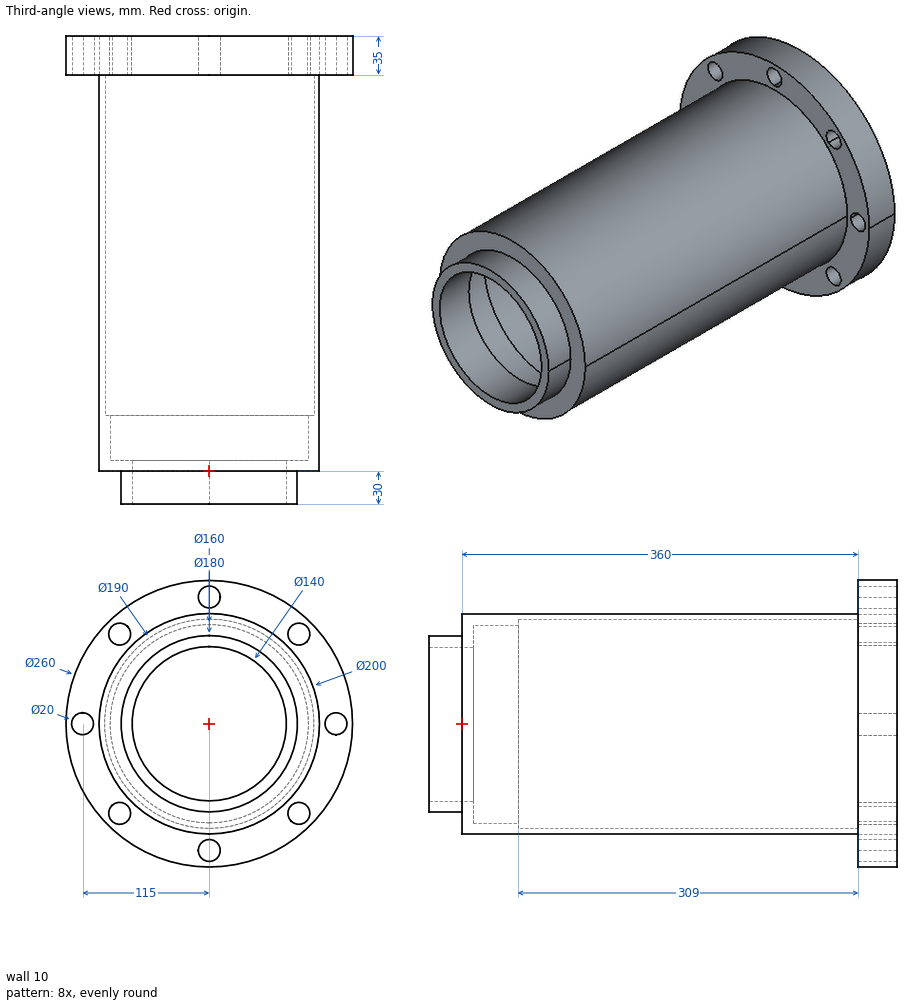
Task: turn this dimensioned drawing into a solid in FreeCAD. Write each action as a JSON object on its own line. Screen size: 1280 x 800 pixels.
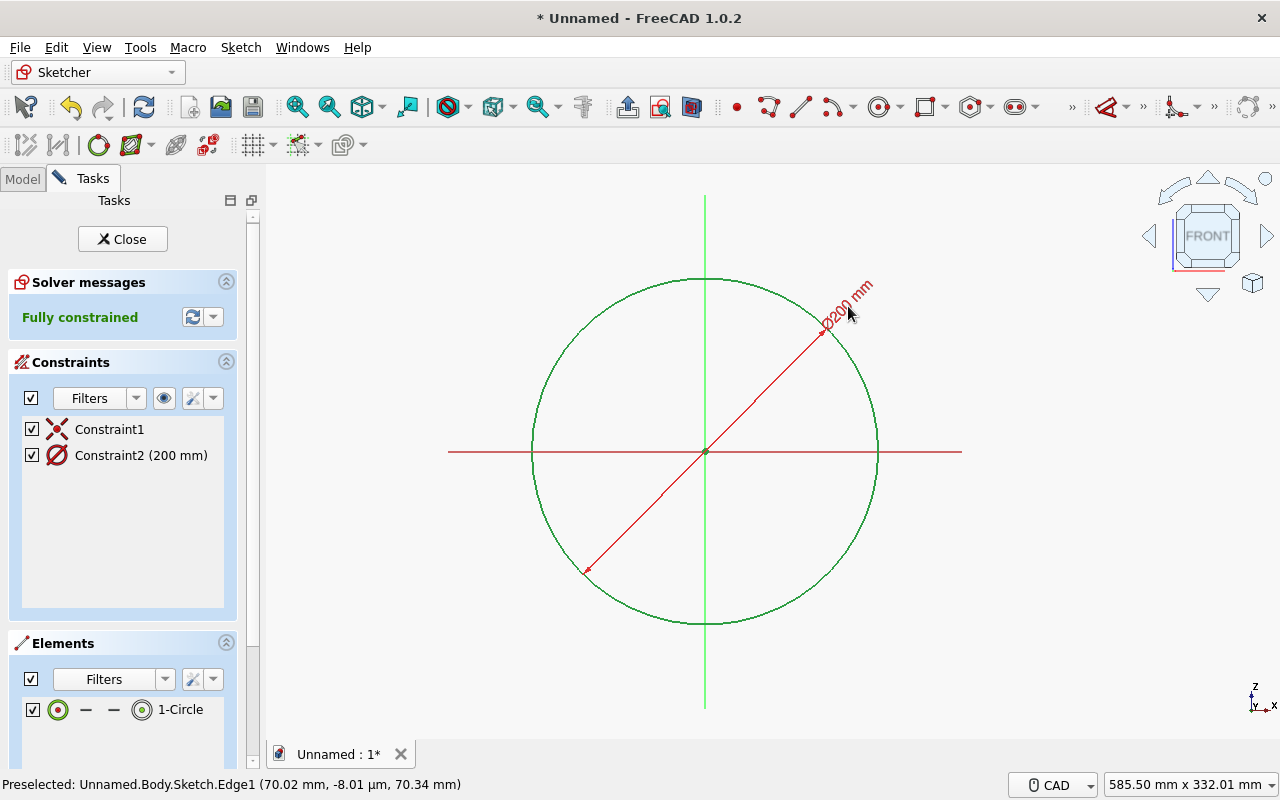
{"action": "left_click", "coordinate": [123, 239]}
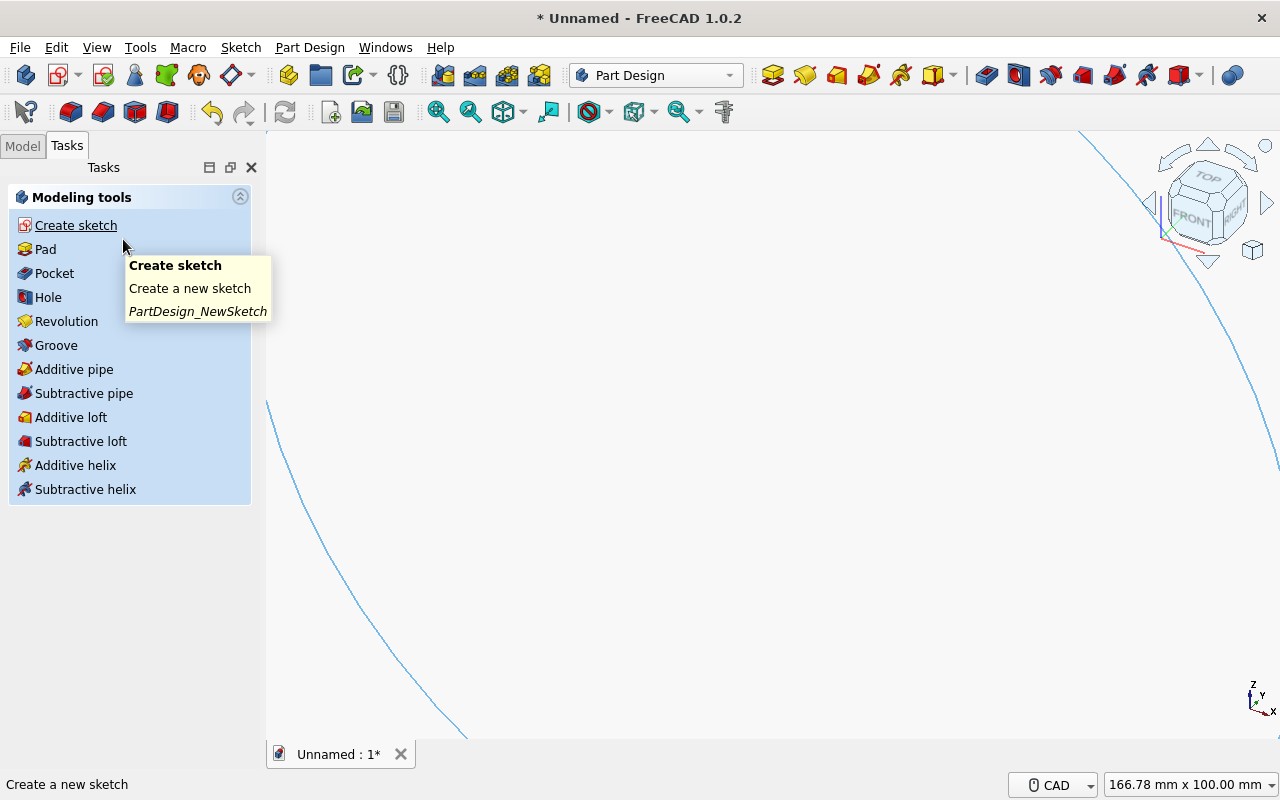
{"action": "left_click", "coordinate": [774, 76]}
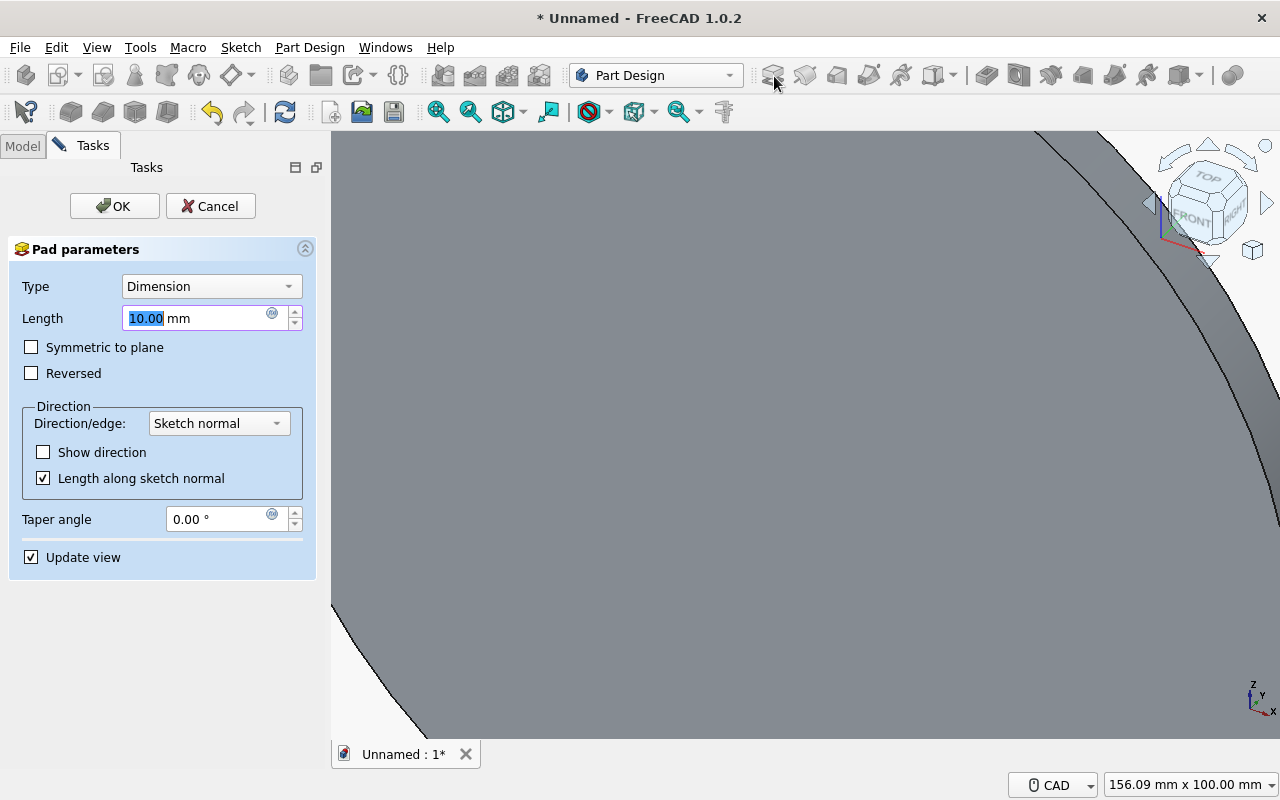
{"action": "type", "text": "360"}
{"action": "key", "text": "Tab"}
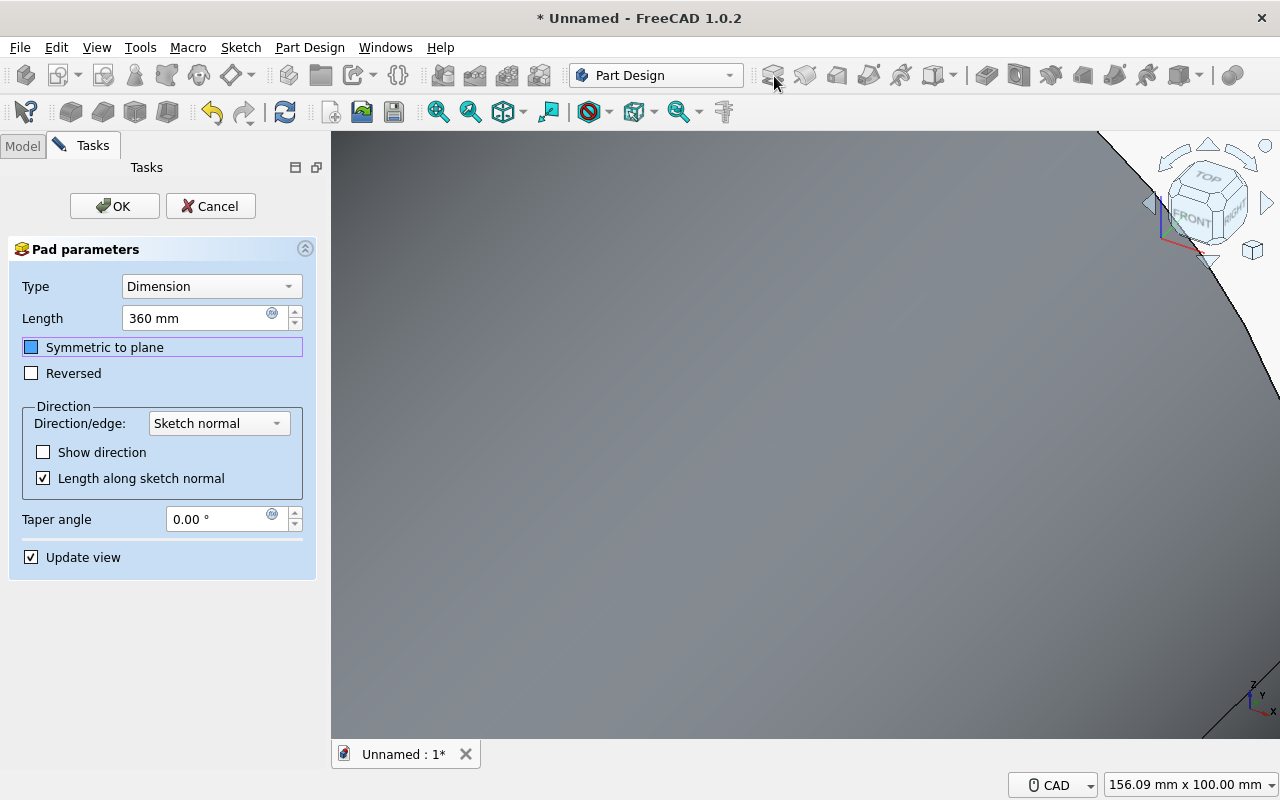
{"action": "left_click", "coordinate": [30, 373]}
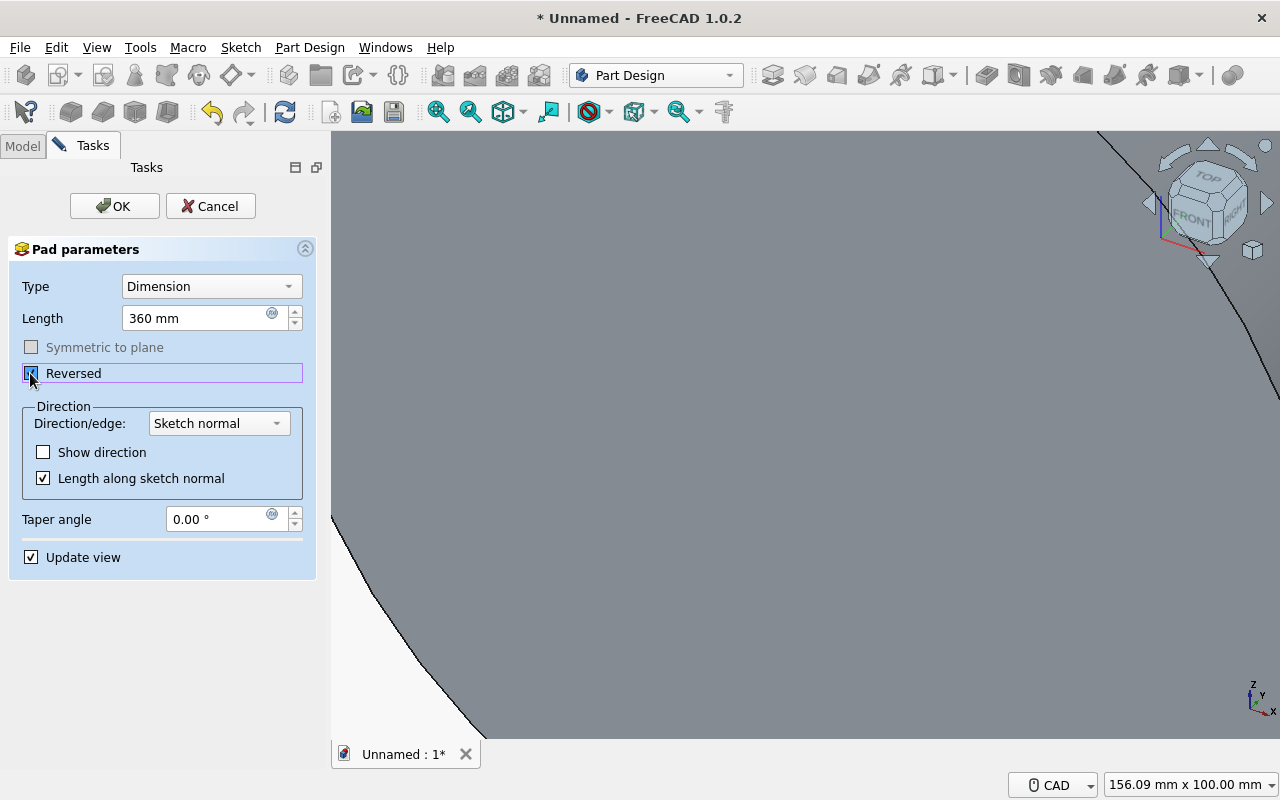
{"action": "left_click", "coordinate": [115, 206]}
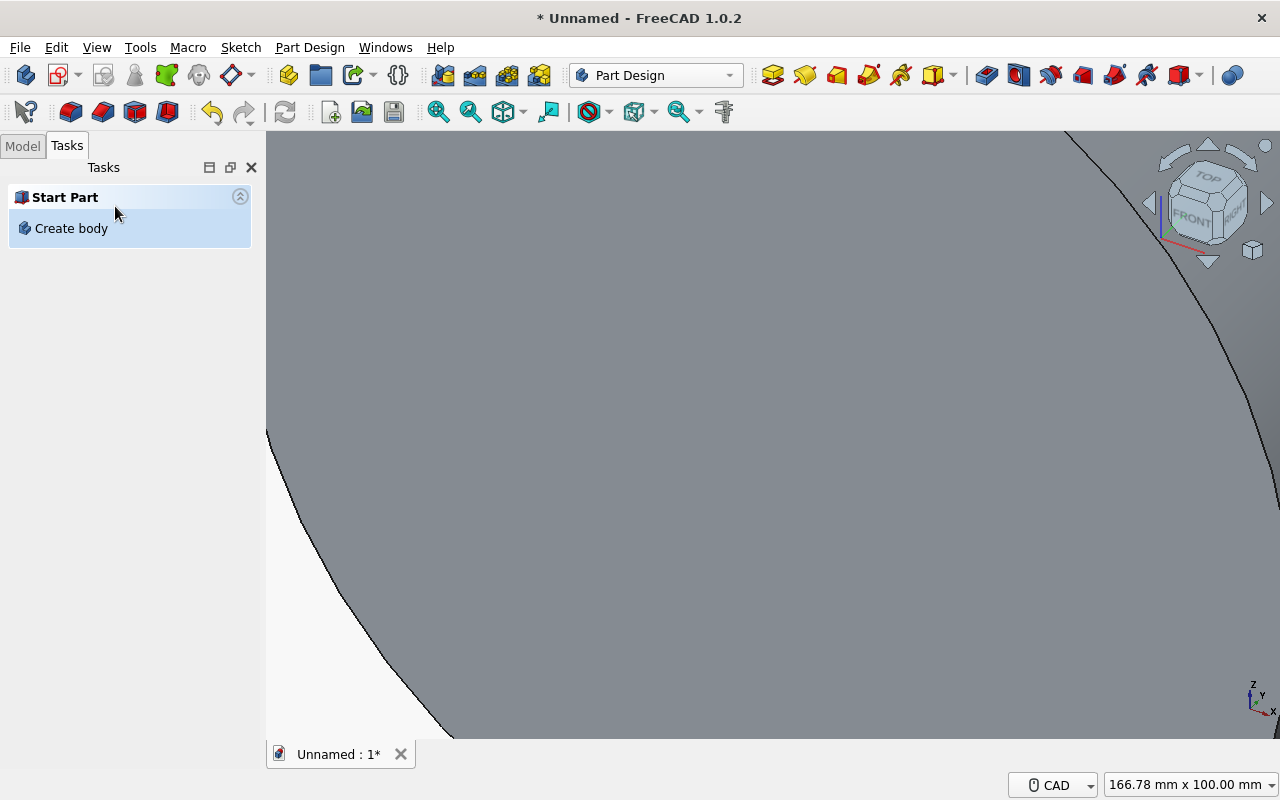
{"action": "left_click", "coordinate": [440, 112]}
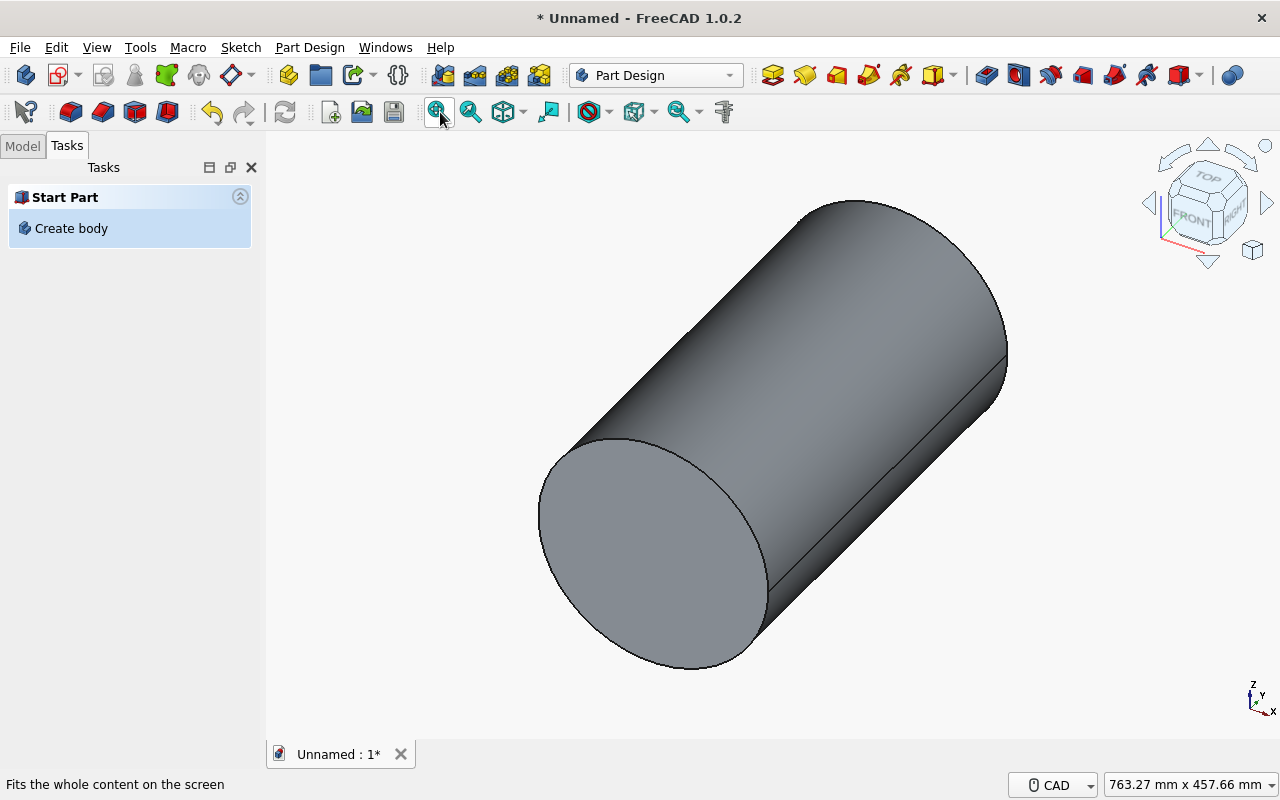
{"action": "key", "text": "0"}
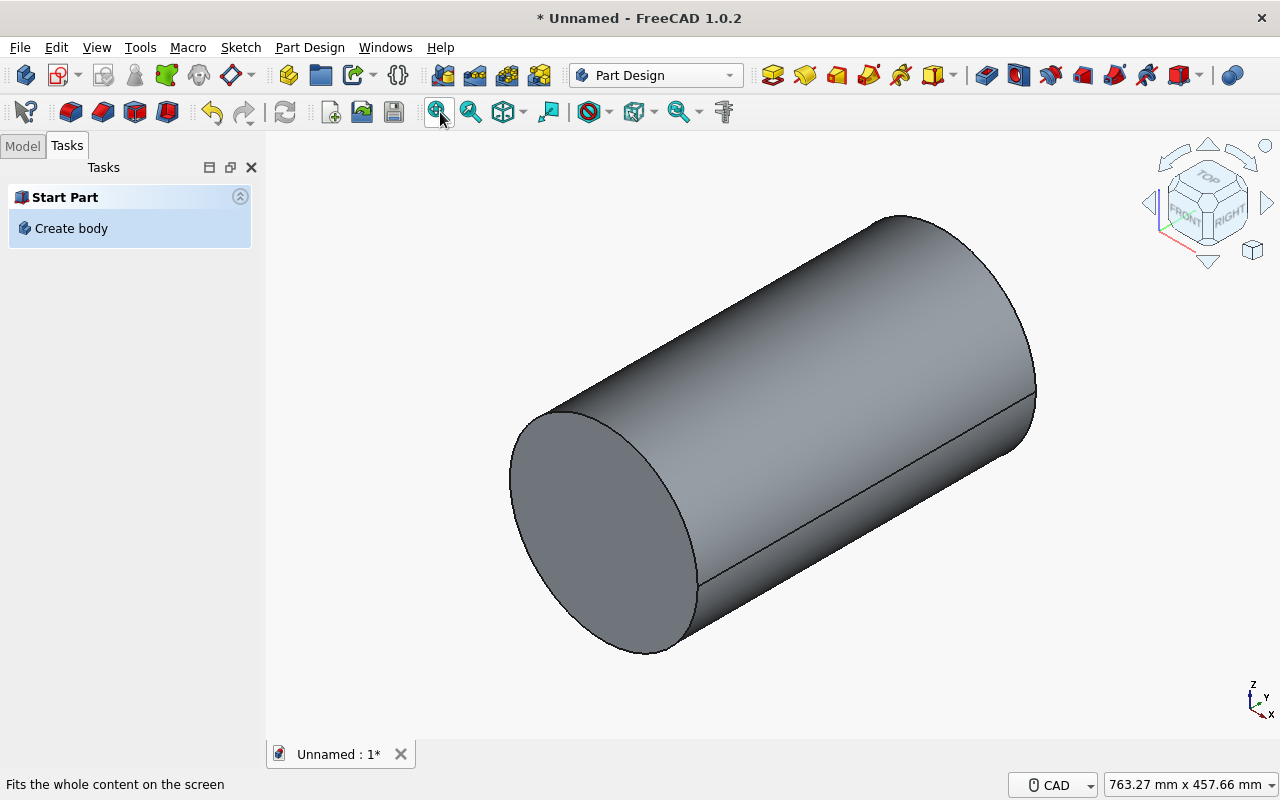
{"action": "key", "text": "2"}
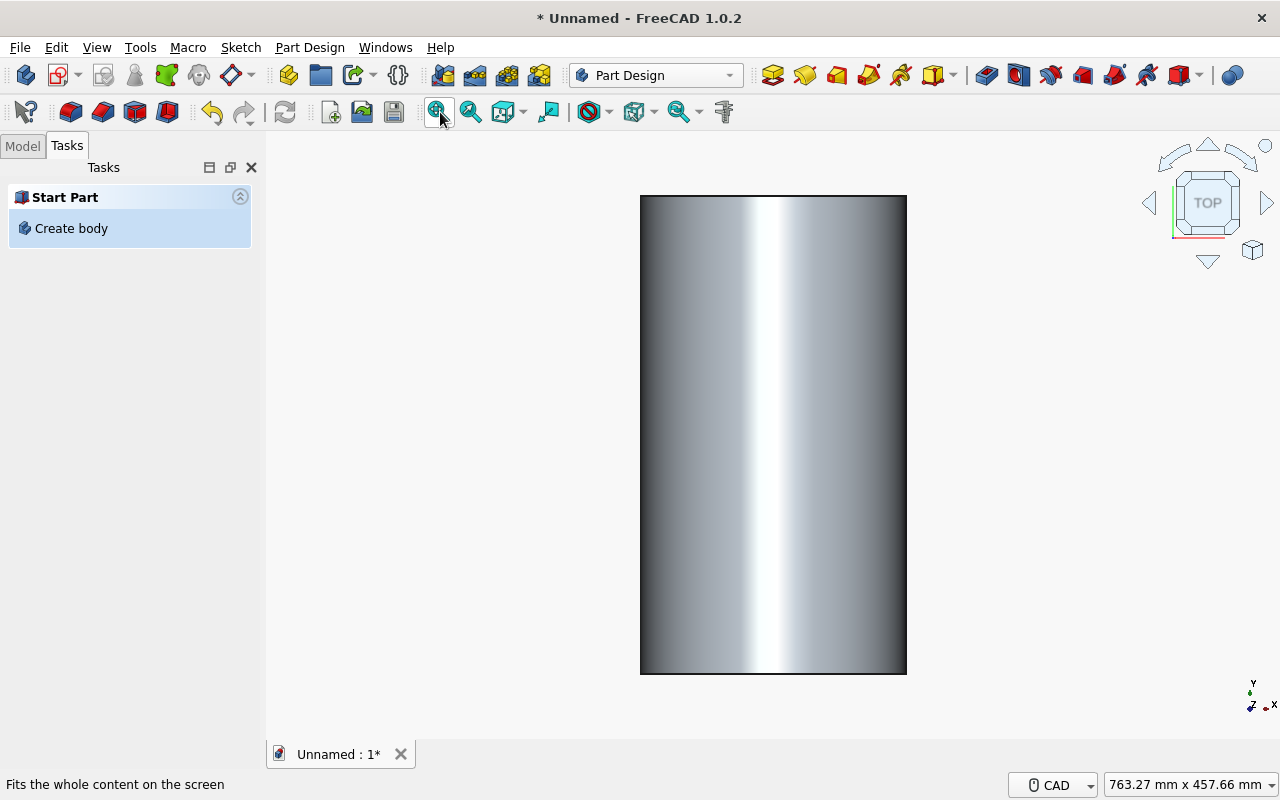
{"action": "key", "text": "1"}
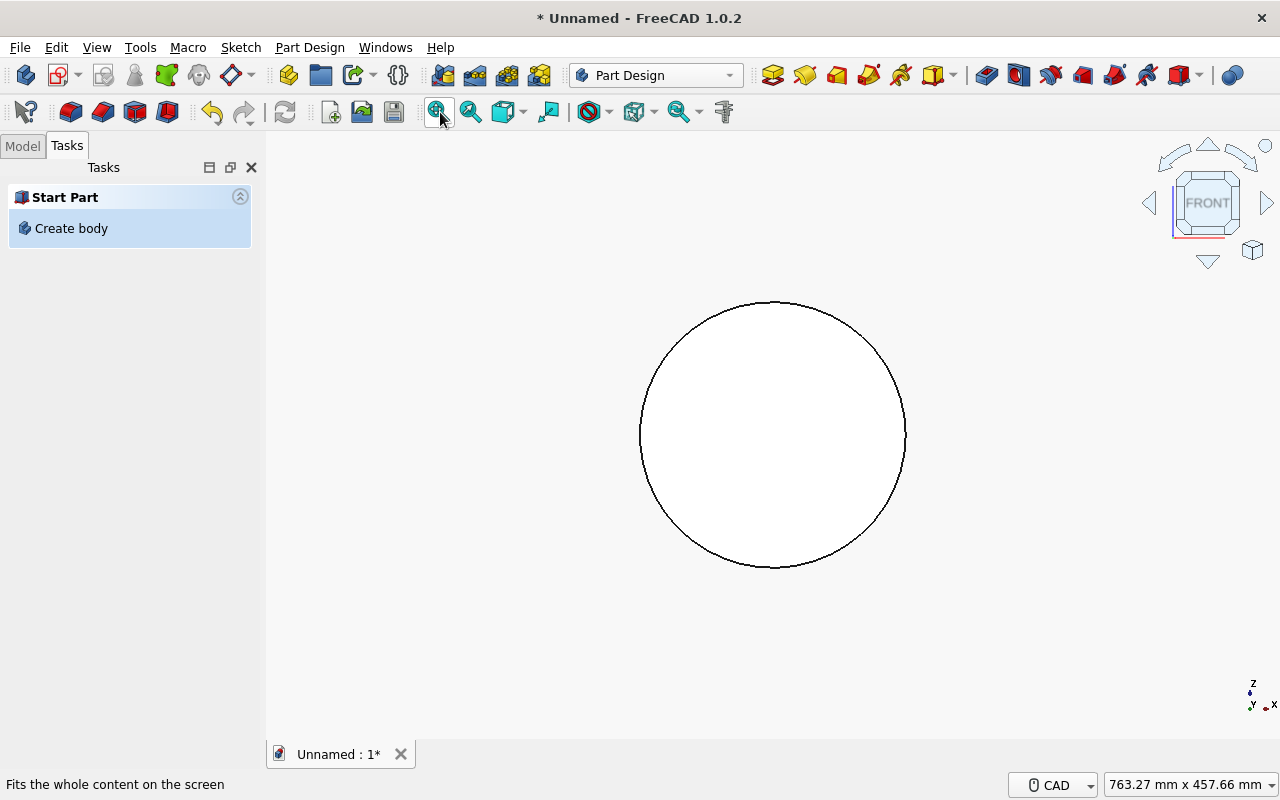
{"action": "key", "text": "v f"}